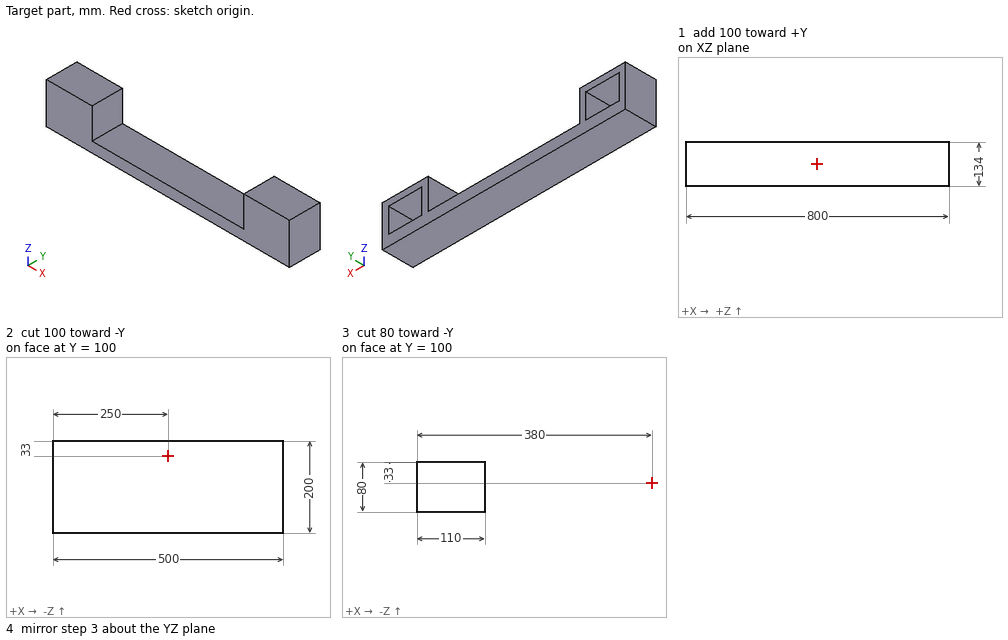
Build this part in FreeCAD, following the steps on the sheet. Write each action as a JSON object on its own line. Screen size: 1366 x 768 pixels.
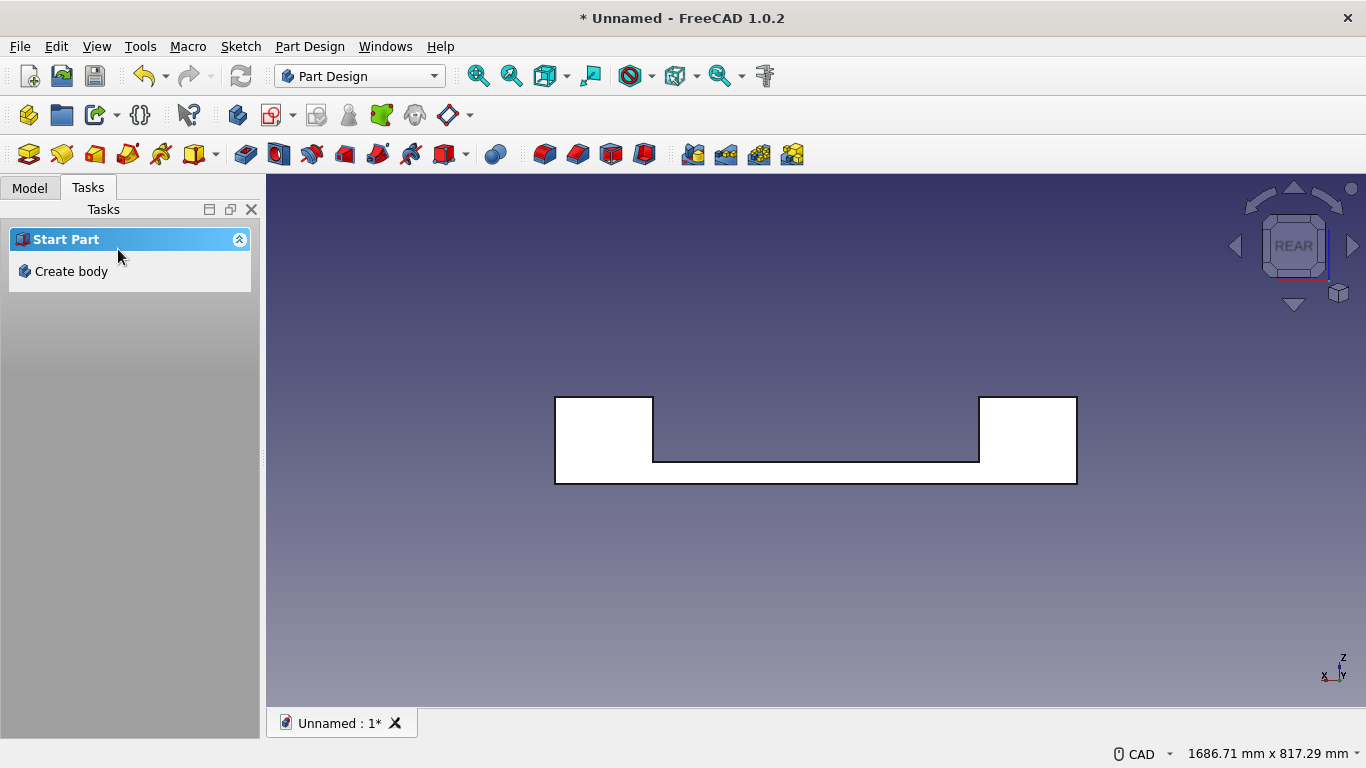
{"action": "left_click", "coordinate": [1040, 440]}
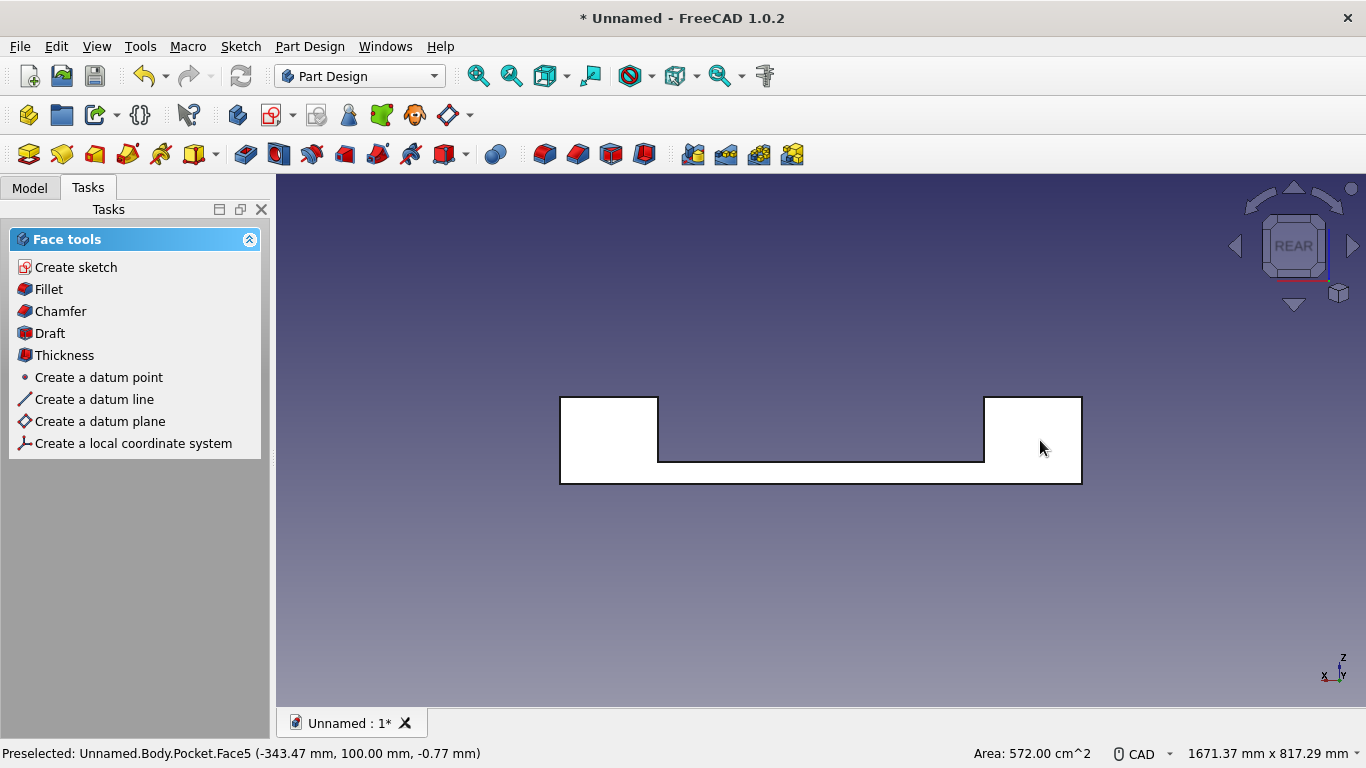
{"action": "left_click", "coordinate": [270, 116]}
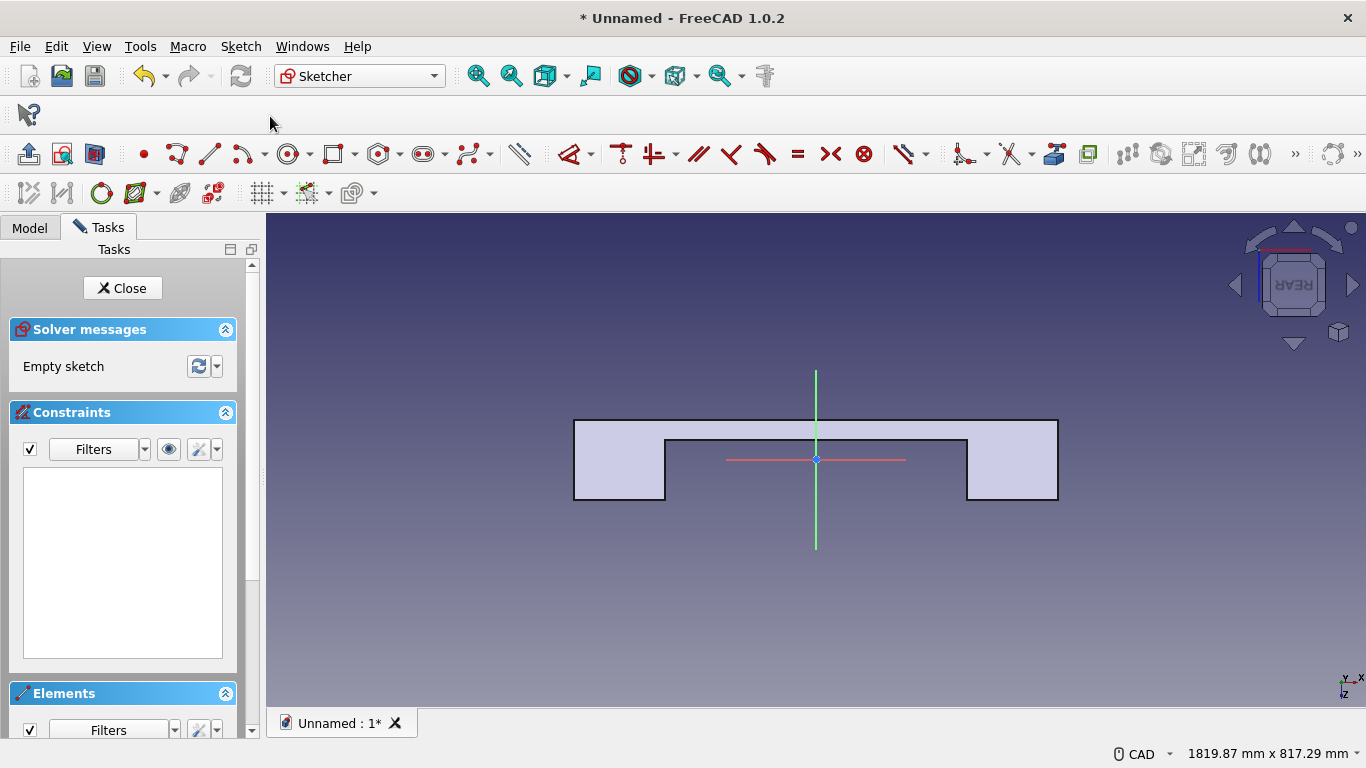
{"action": "scroll", "coordinate": [594, 465], "scroll_direction": "up", "scroll_amount": 9}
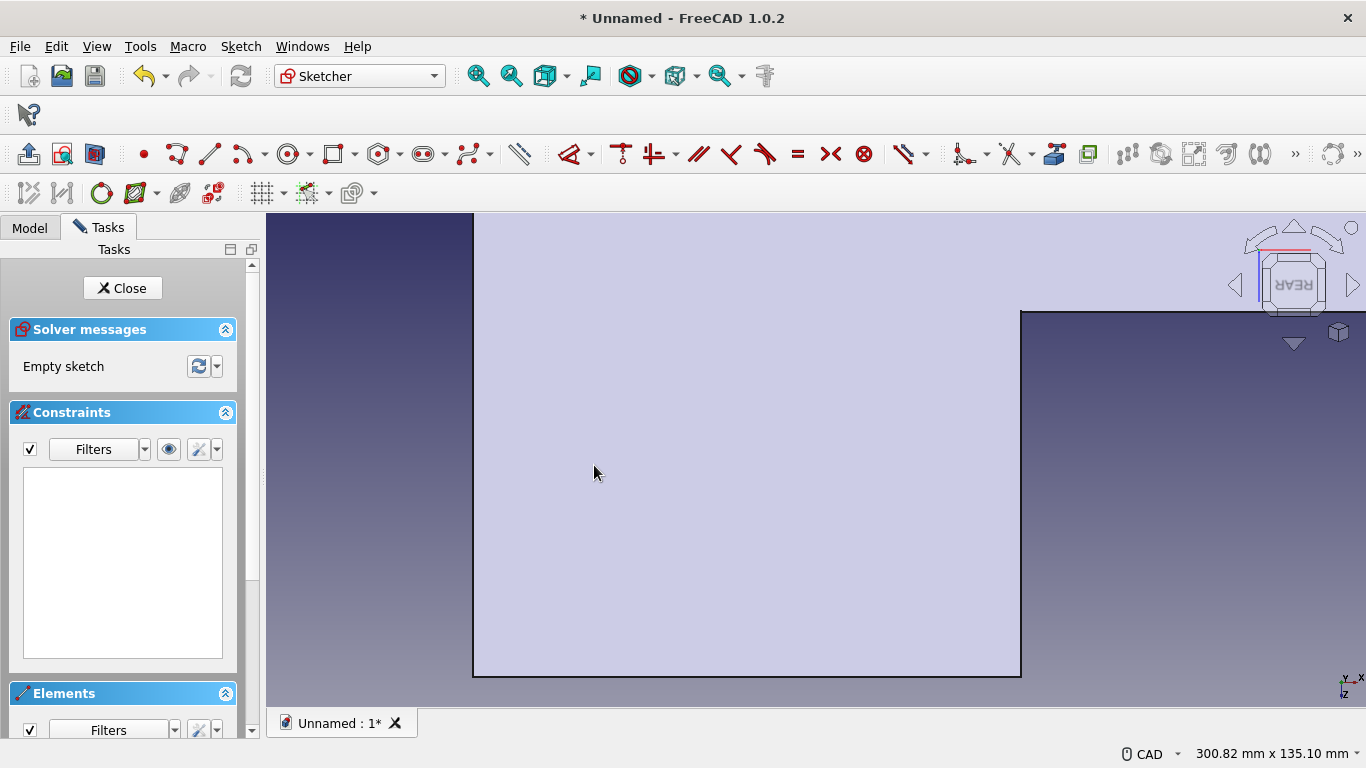
{"action": "left_click", "coordinate": [332, 154]}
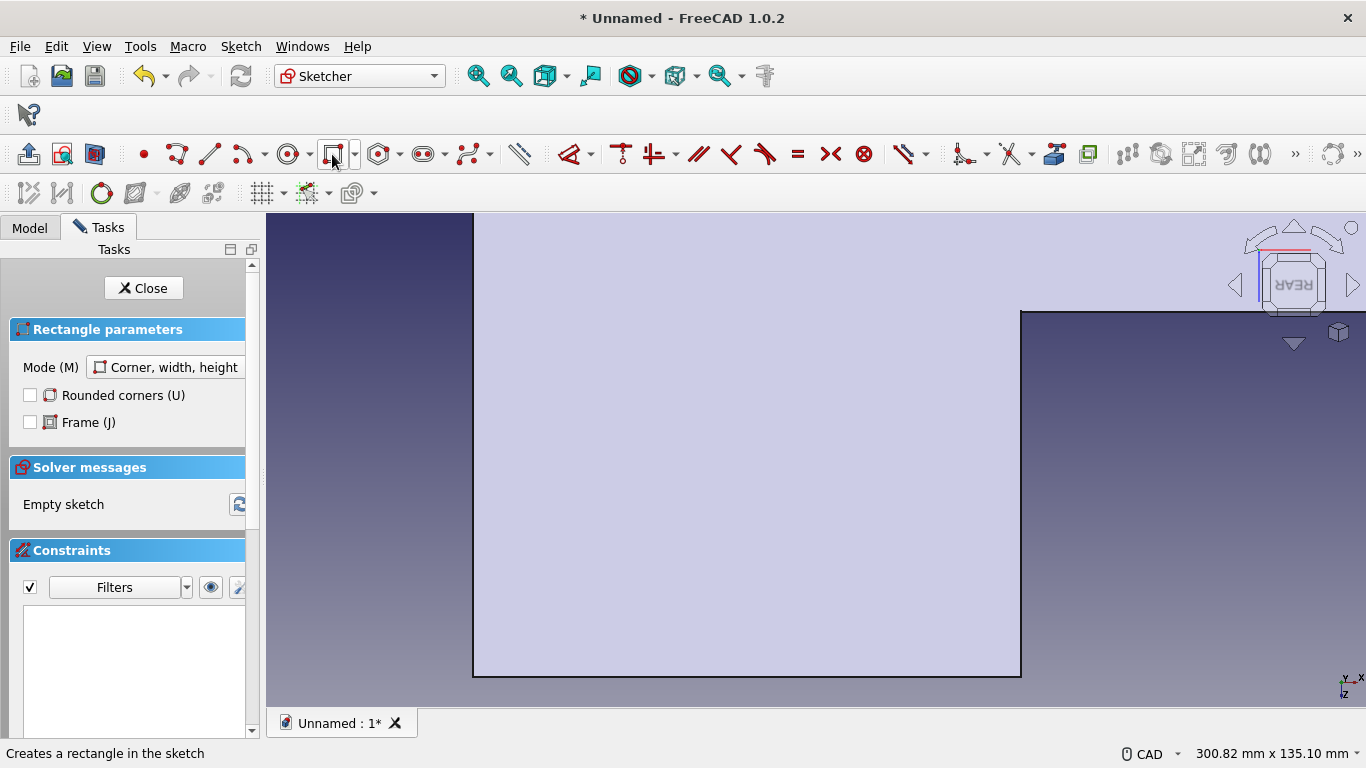
{"action": "left_click", "coordinate": [546, 312]}
{"action": "mouse_move", "coordinate": [948, 604]}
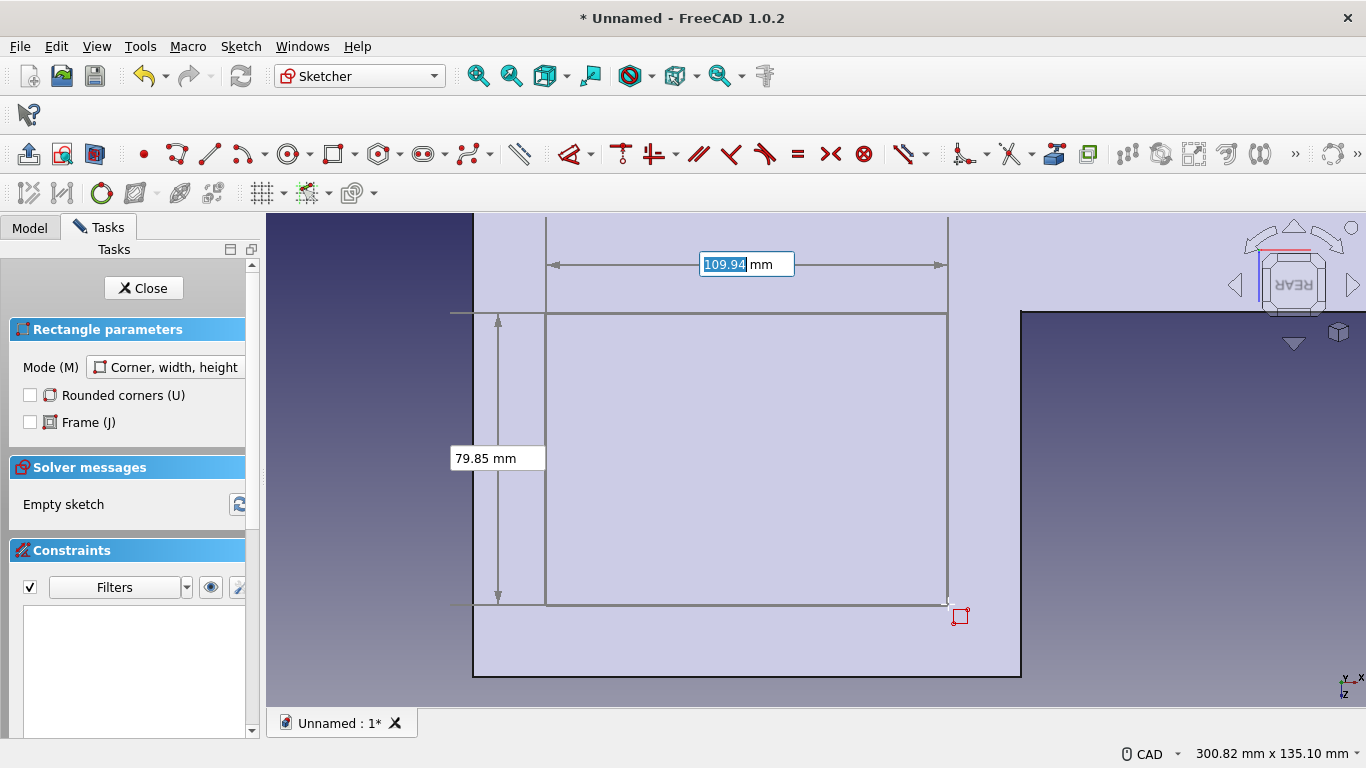
{"action": "type", "text": "110"}
{"action": "key", "text": "Tab"}
{"action": "type", "text": "80"}
{"action": "key", "text": "Return"}
{"action": "key", "text": "Escape"}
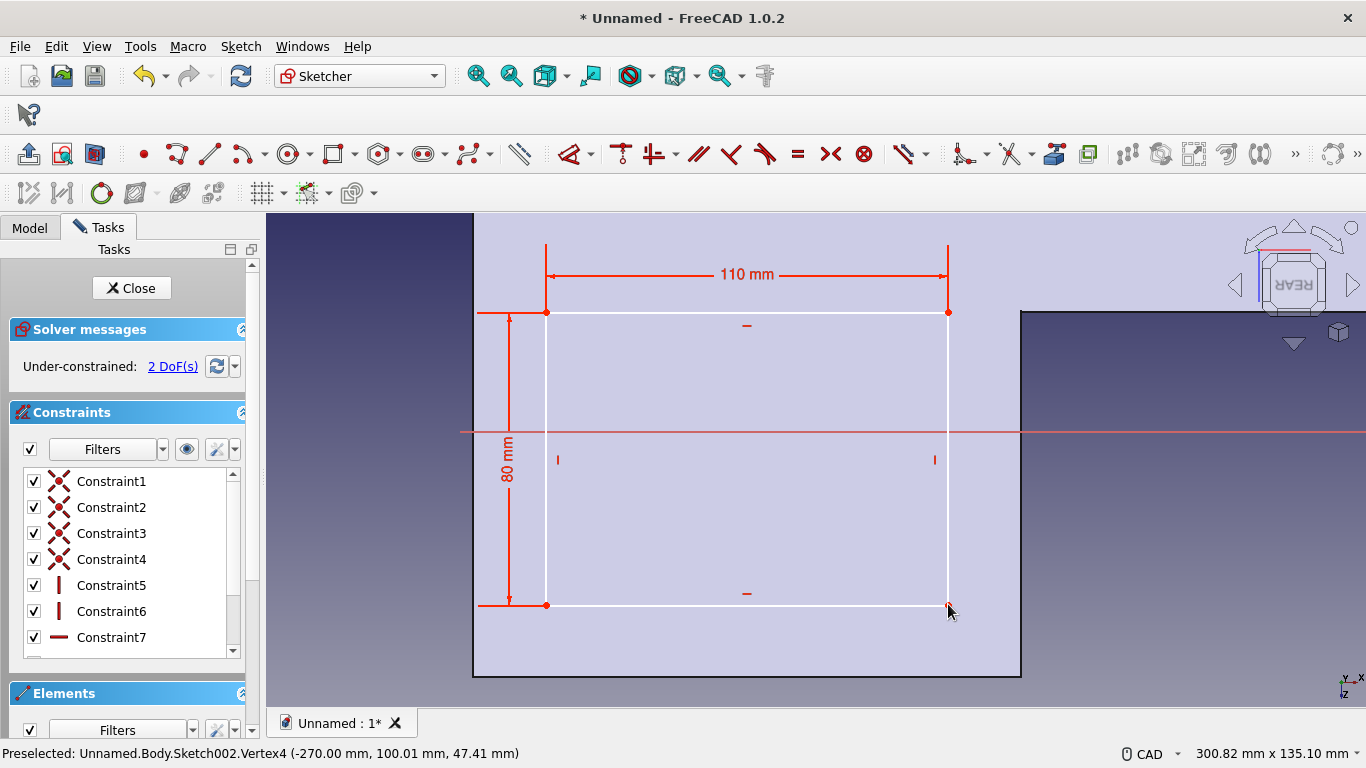
{"action": "left_click", "coordinate": [568, 154]}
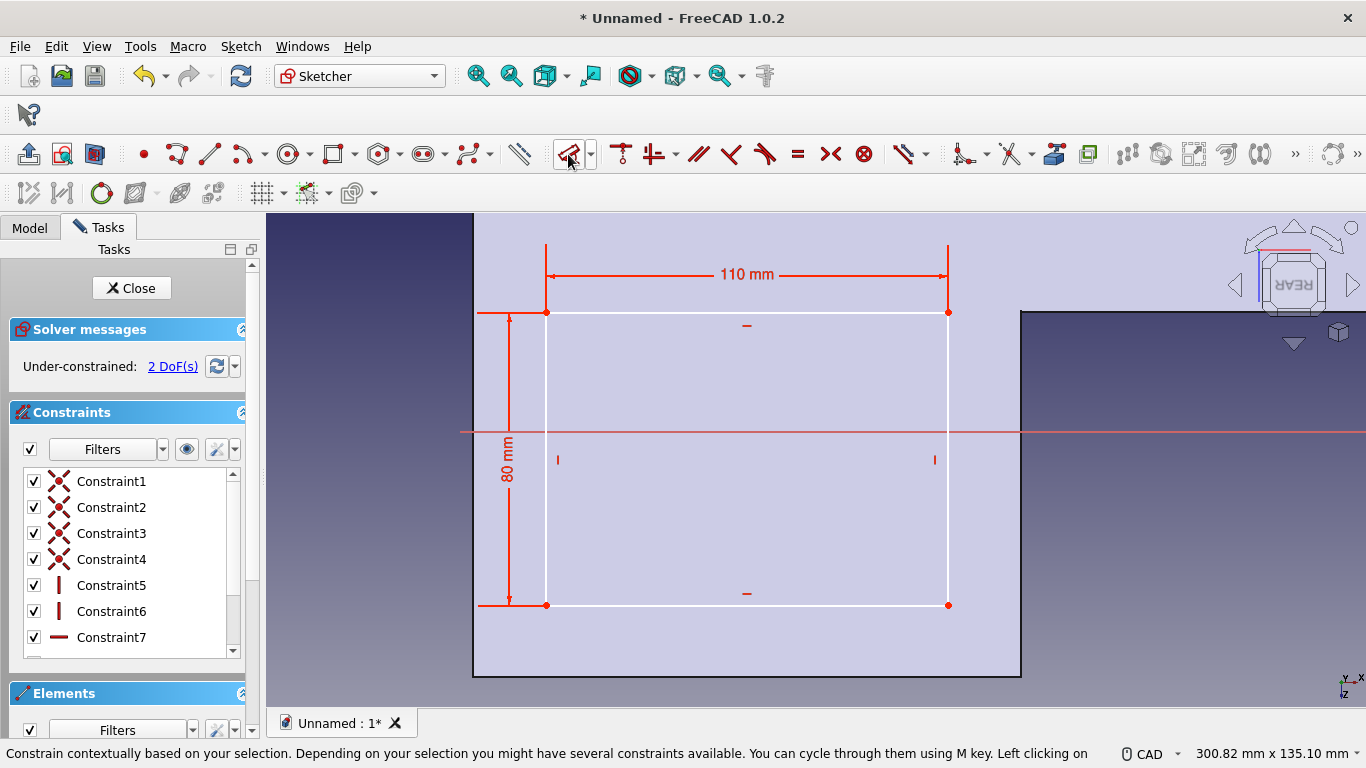
{"action": "left_click", "coordinate": [546, 313]}
{"action": "left_click", "coordinate": [512, 373]}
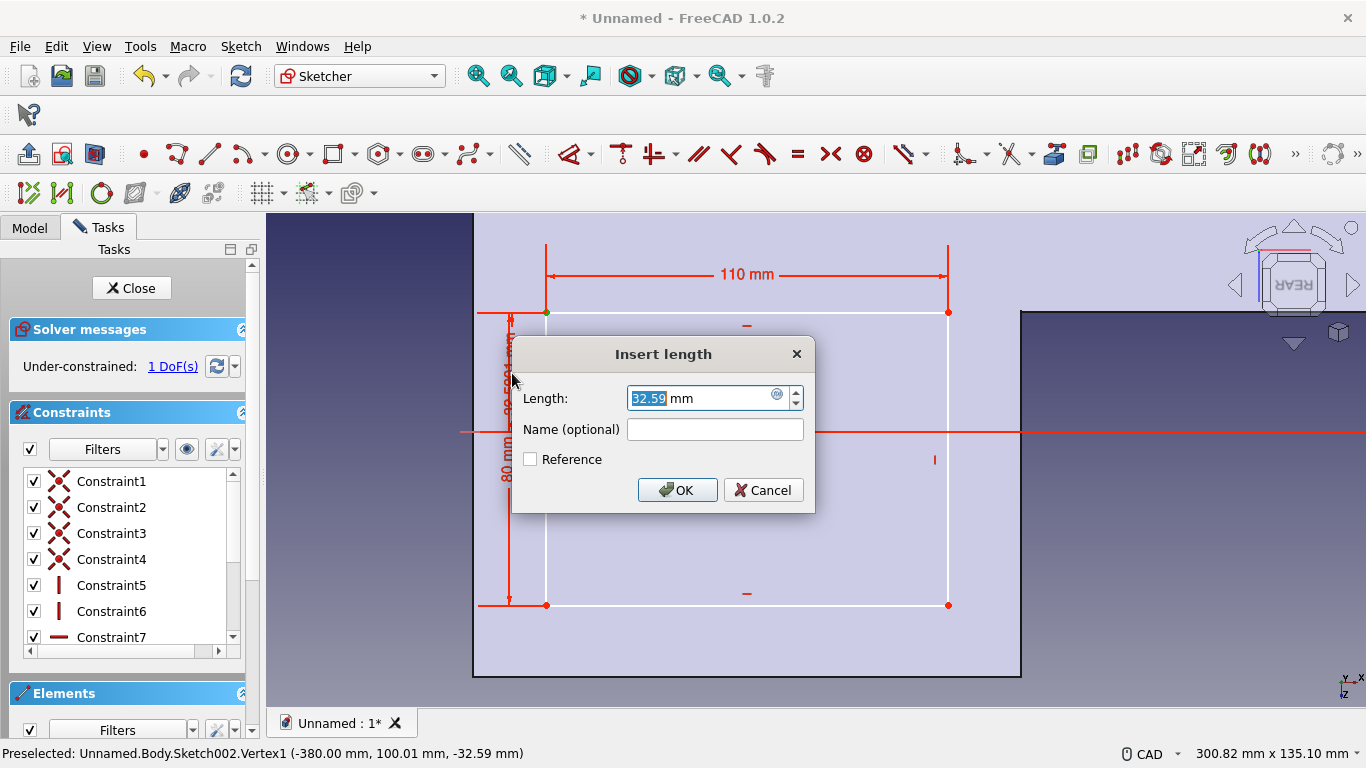
{"action": "type", "text": "33"}
{"action": "key", "text": "Return"}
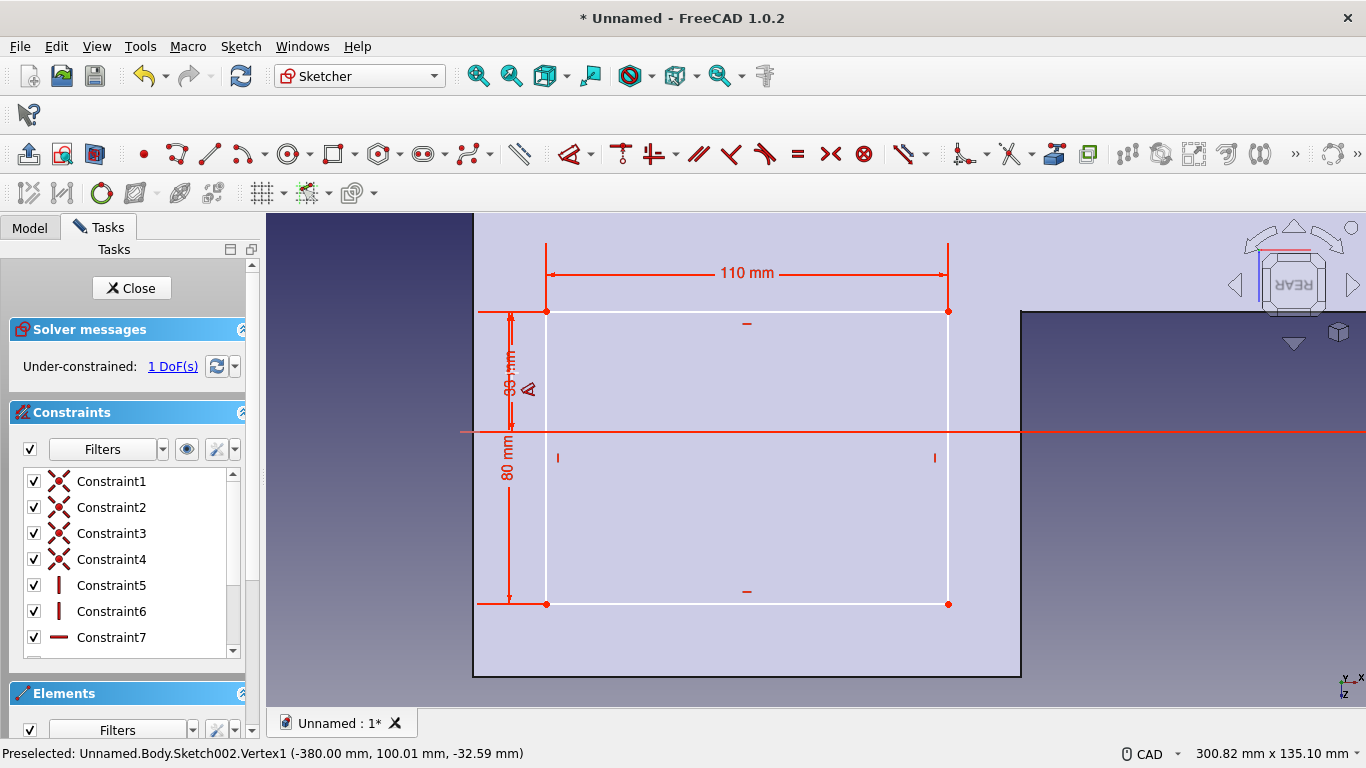
{"action": "left_click", "coordinate": [546, 312]}
{"action": "left_click", "coordinate": [874, 278]}